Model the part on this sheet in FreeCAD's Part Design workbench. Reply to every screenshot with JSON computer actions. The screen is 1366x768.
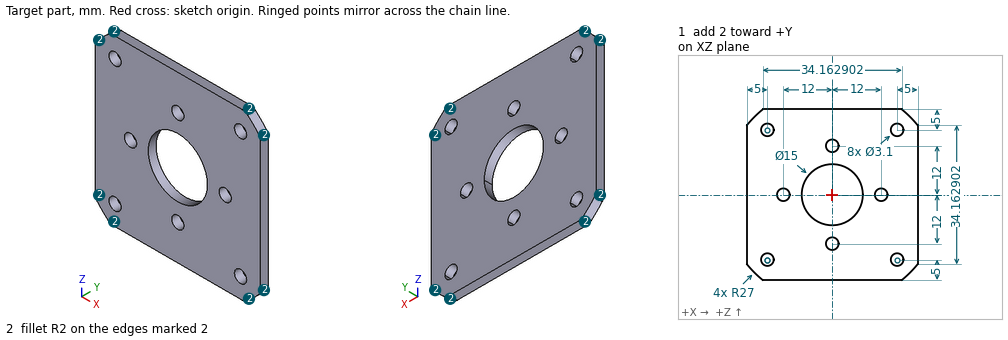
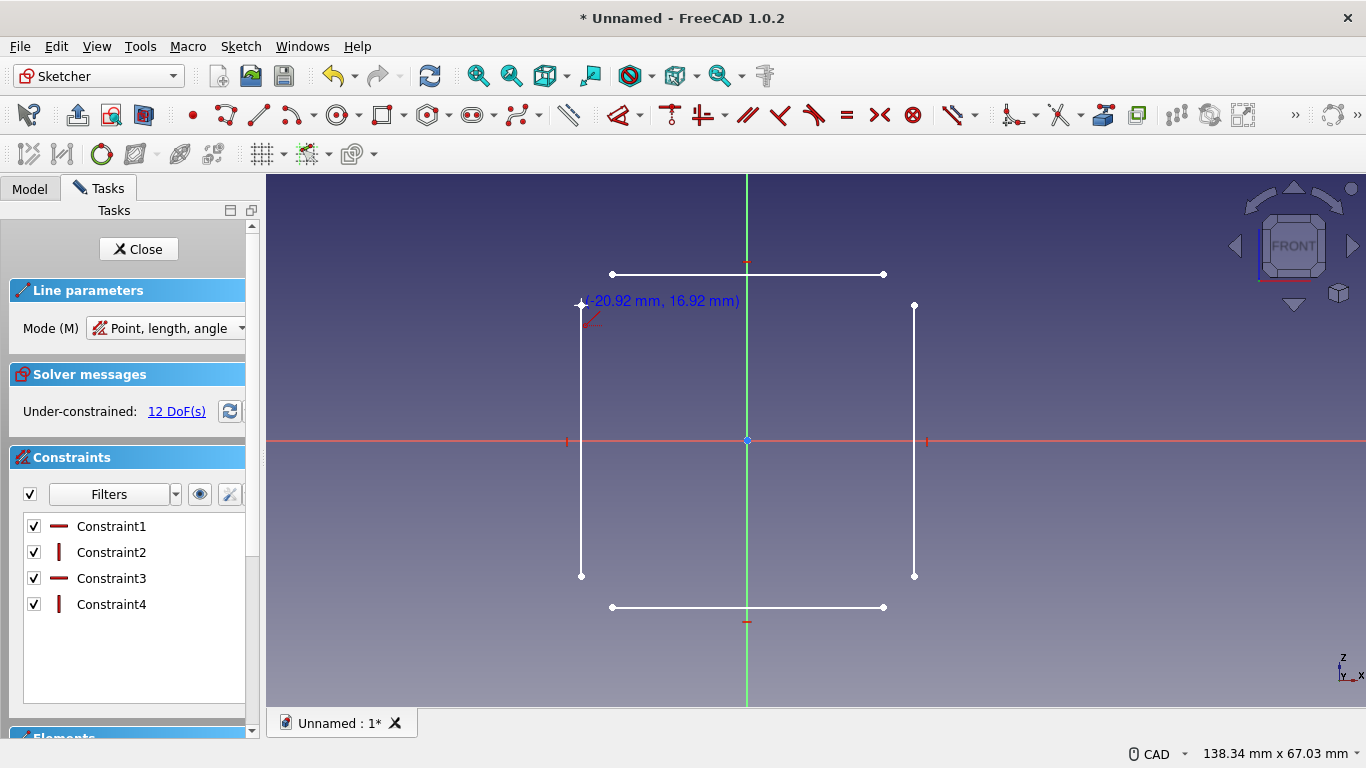
{"action": "left_click", "coordinate": [314, 116]}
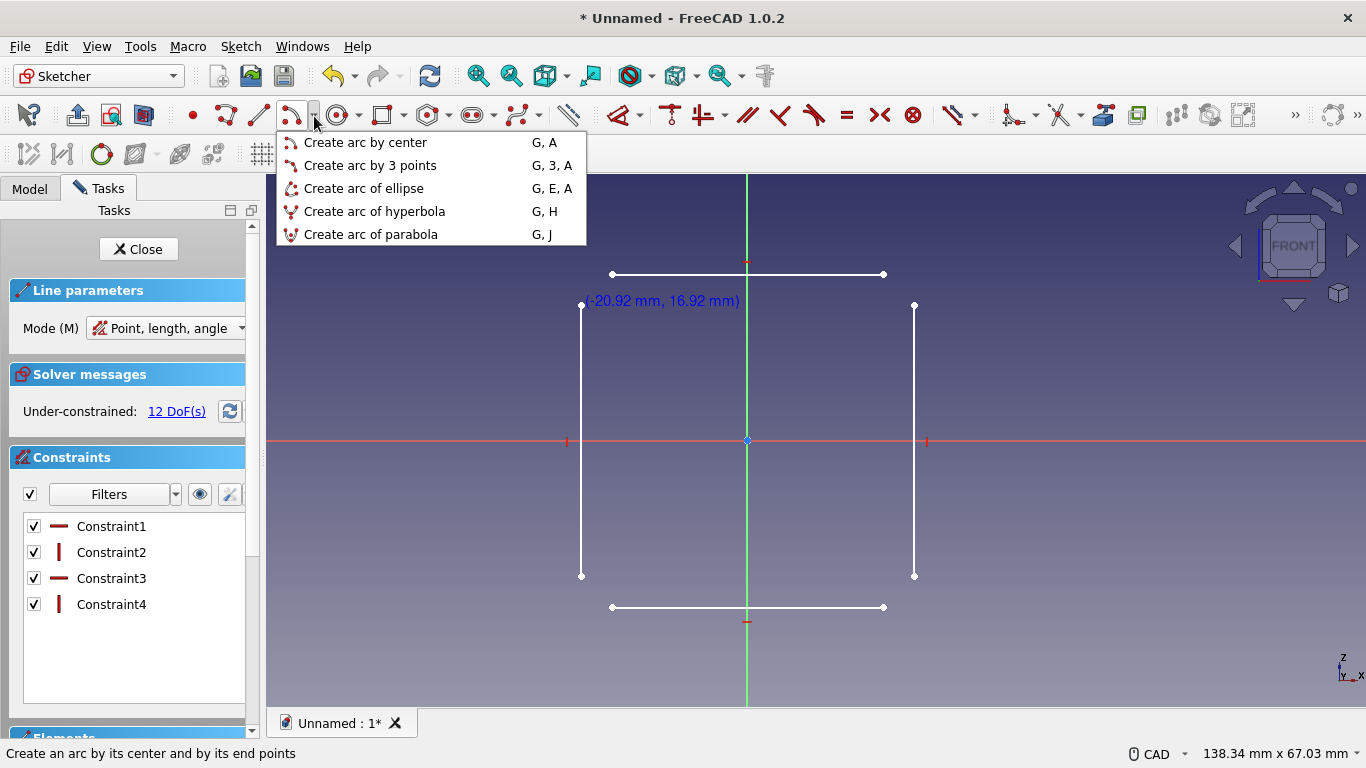
{"action": "left_click", "coordinate": [432, 166]}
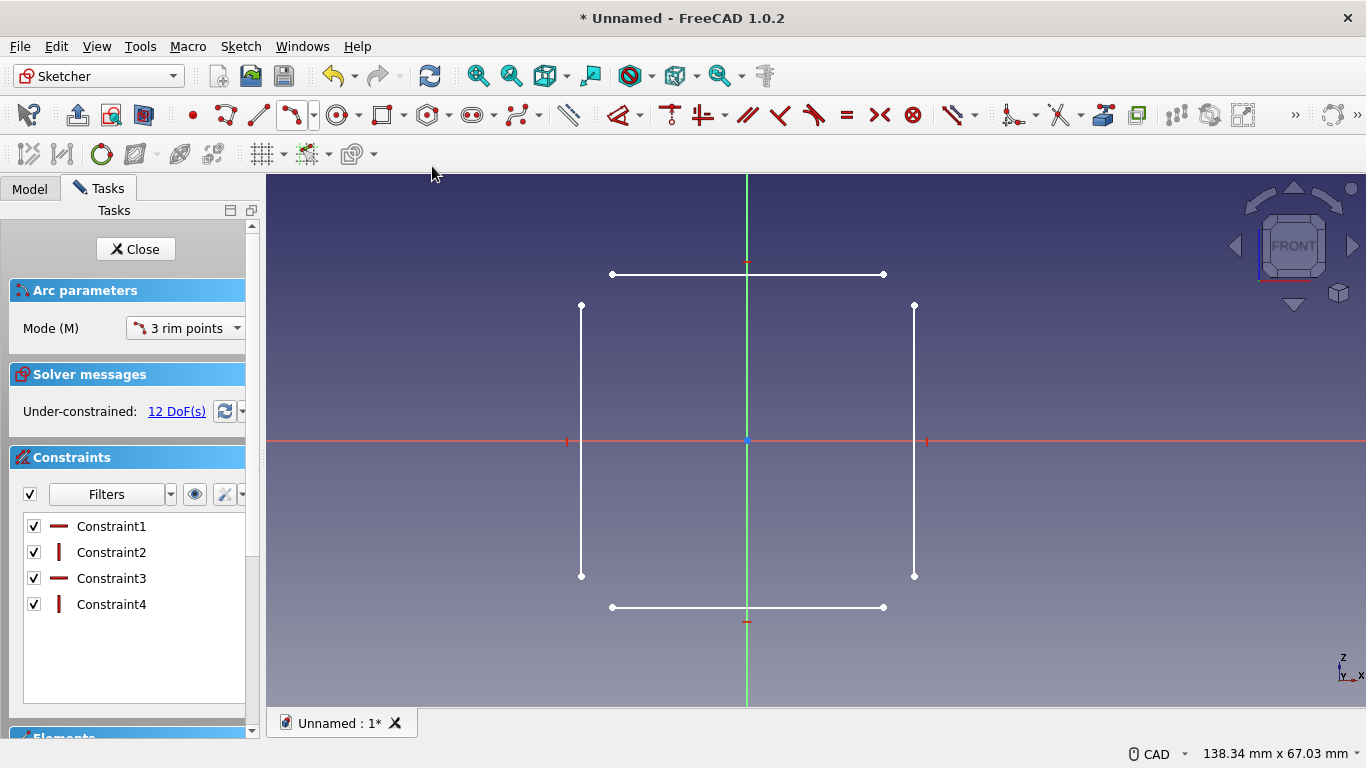
{"action": "left_click", "coordinate": [883, 275]}
{"action": "left_click", "coordinate": [914, 306]}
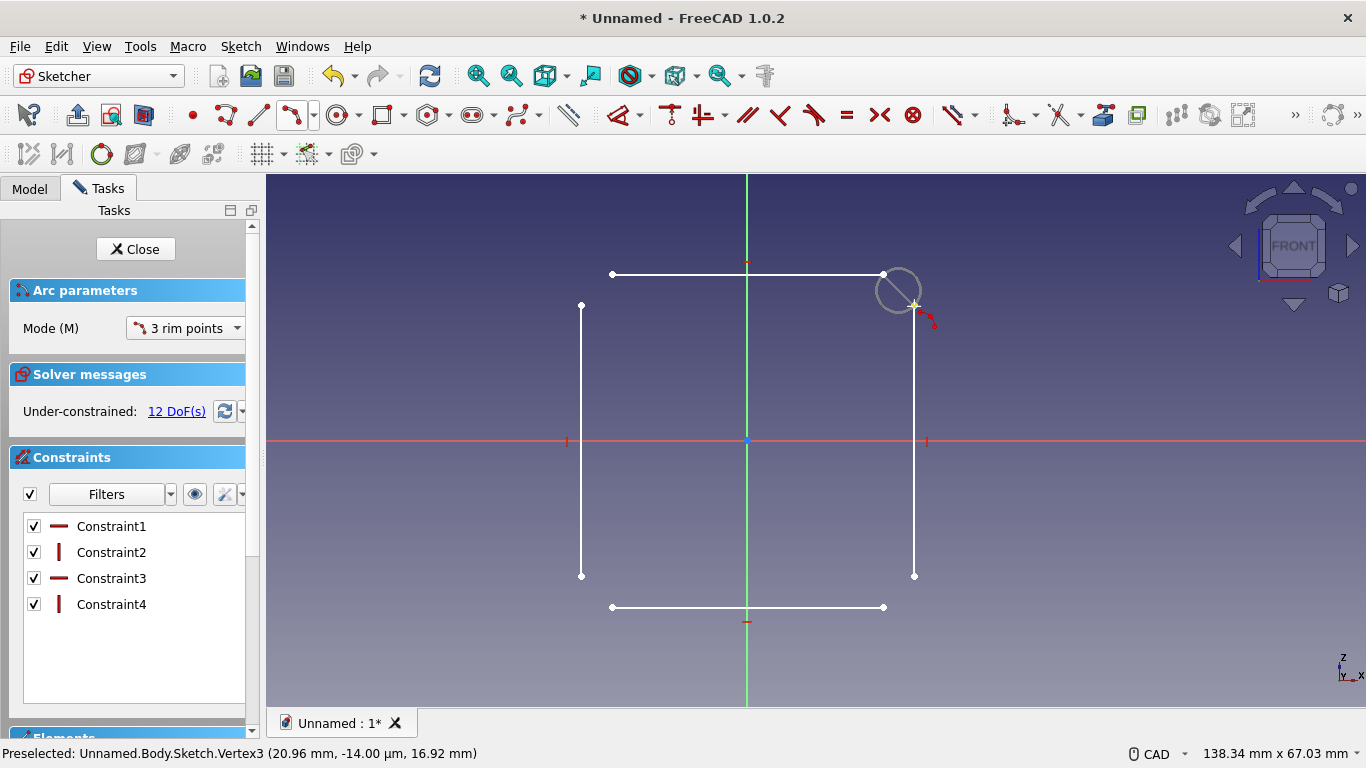
{"action": "scroll", "coordinate": [899, 289], "scroll_direction": "up", "scroll_amount": 14}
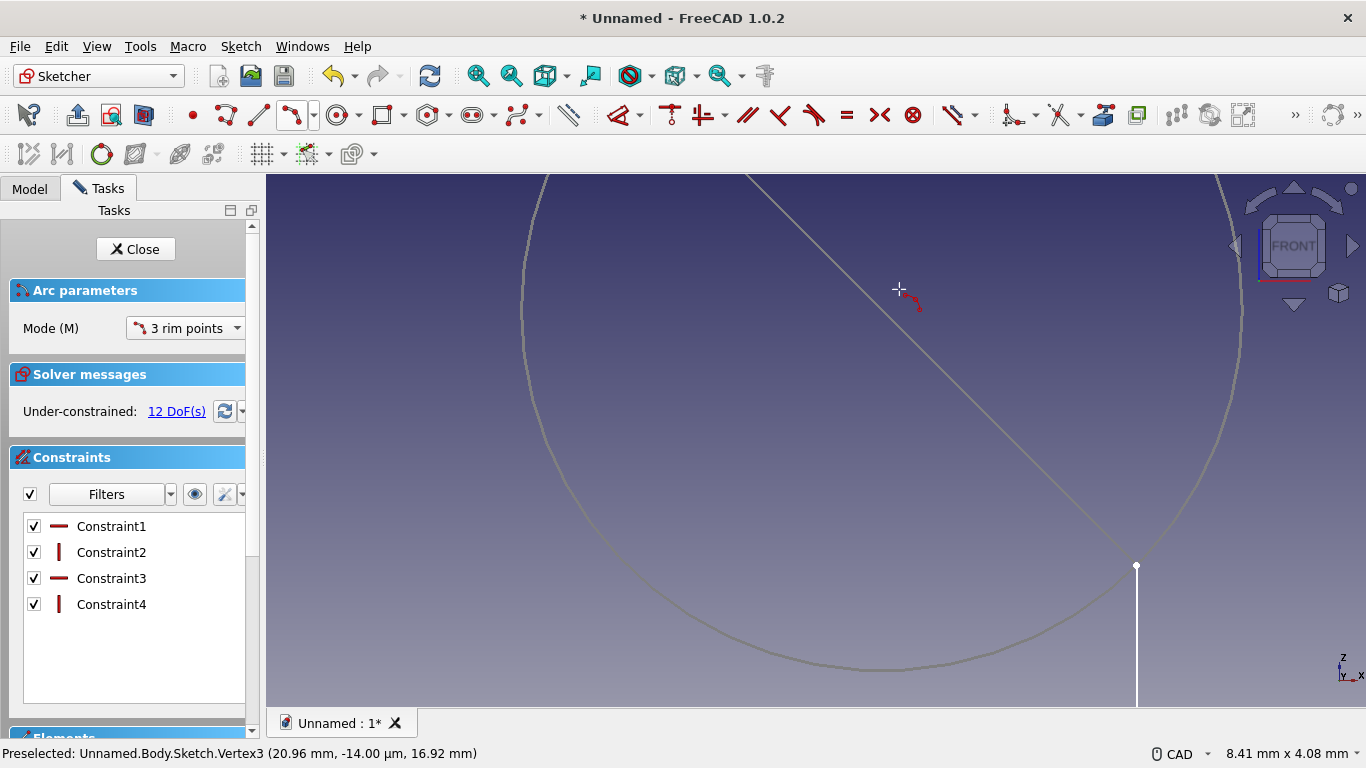
{"action": "left_click", "coordinate": [892, 281]}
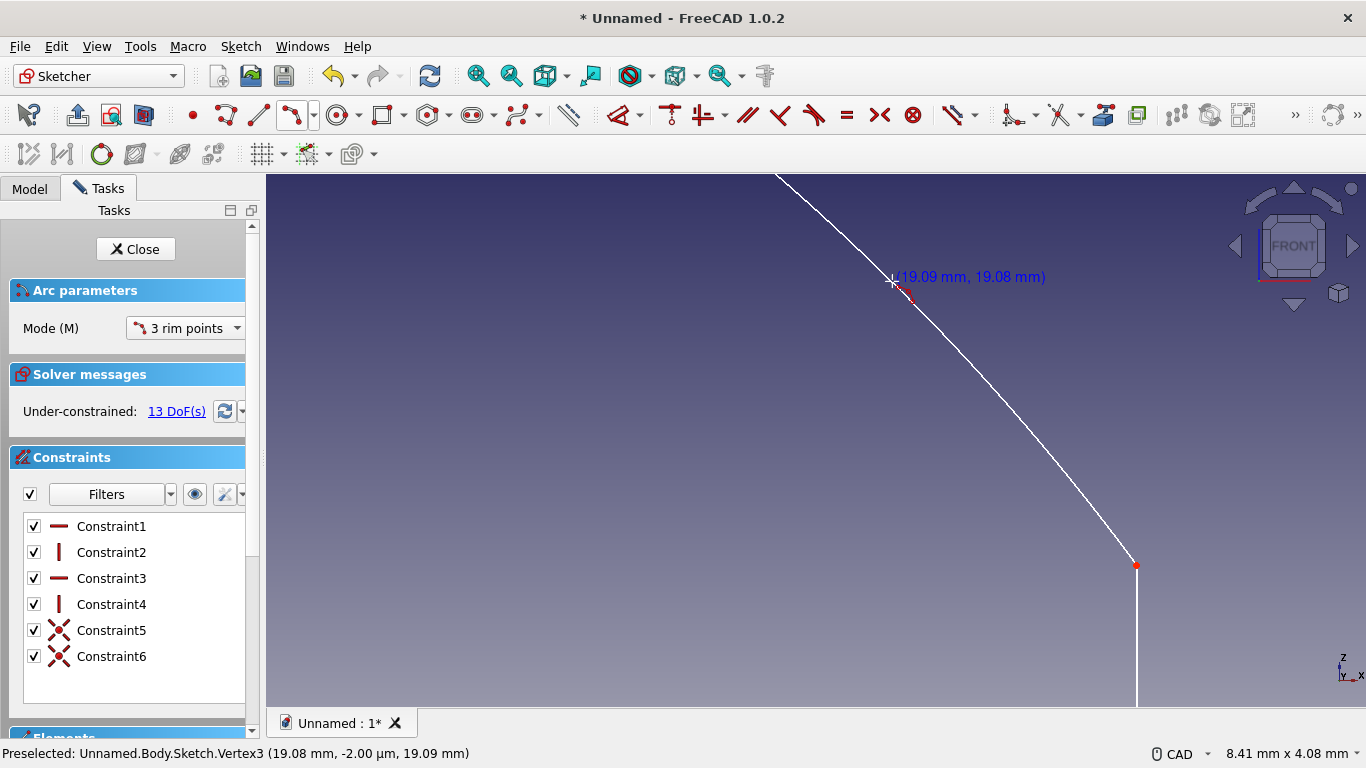
{"action": "scroll", "coordinate": [900, 289], "scroll_direction": "down", "scroll_amount": 14}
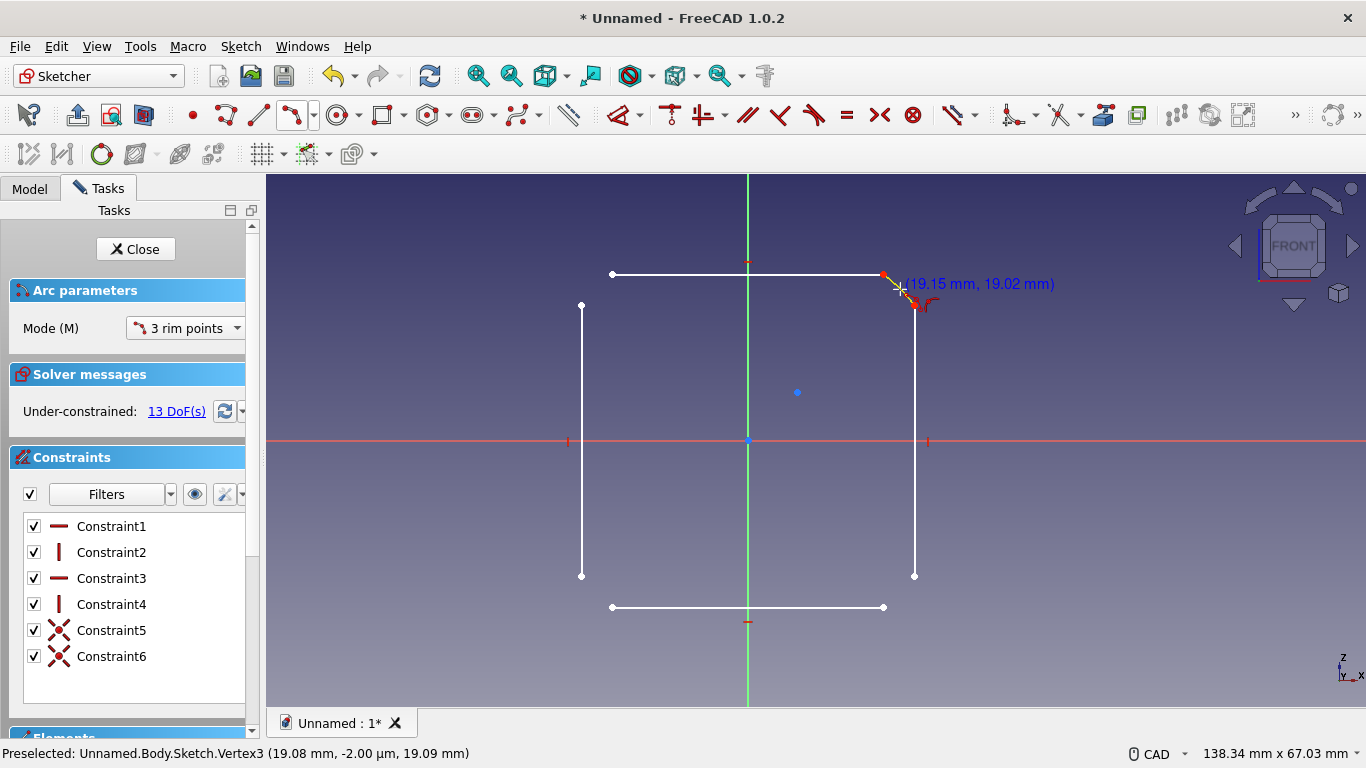
{"action": "left_click", "coordinate": [915, 577]}
{"action": "left_click", "coordinate": [884, 608]}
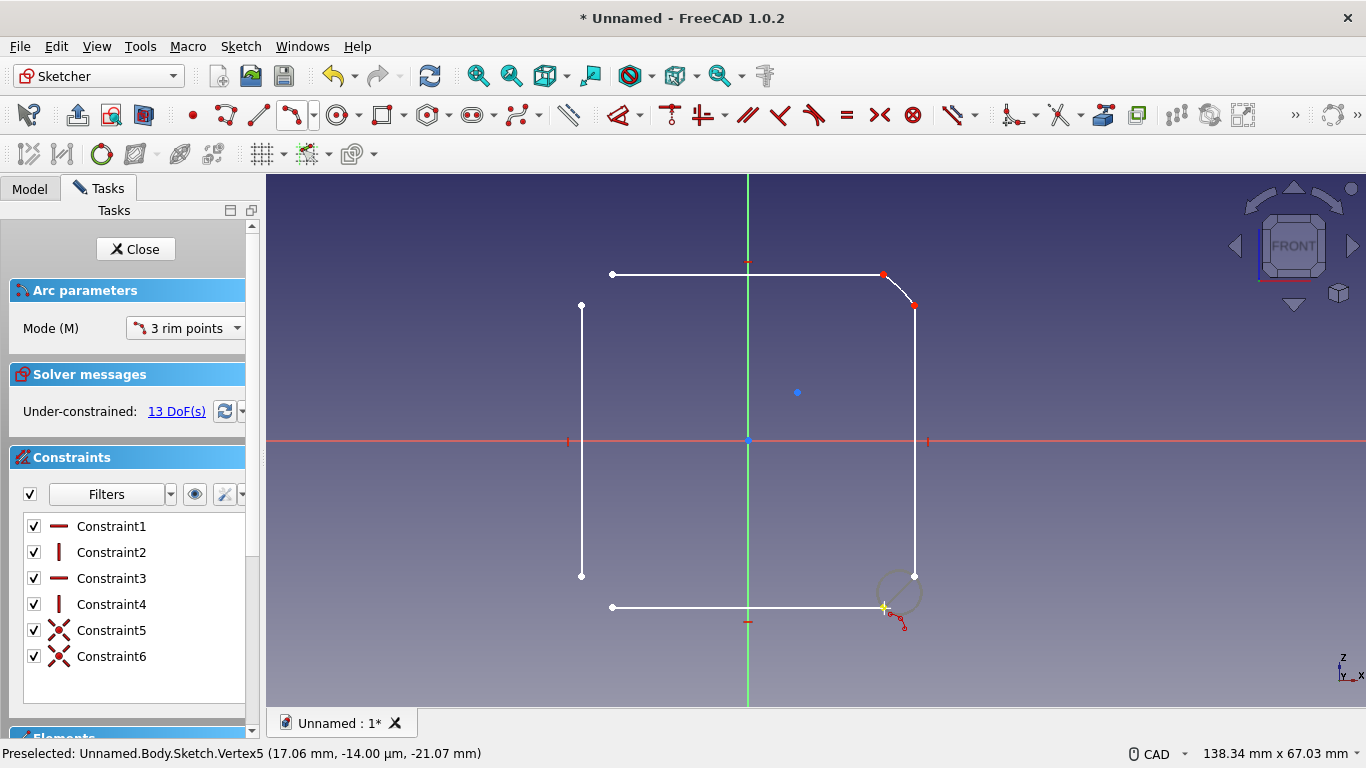
{"action": "scroll", "coordinate": [900, 592], "scroll_direction": "up", "scroll_amount": 14}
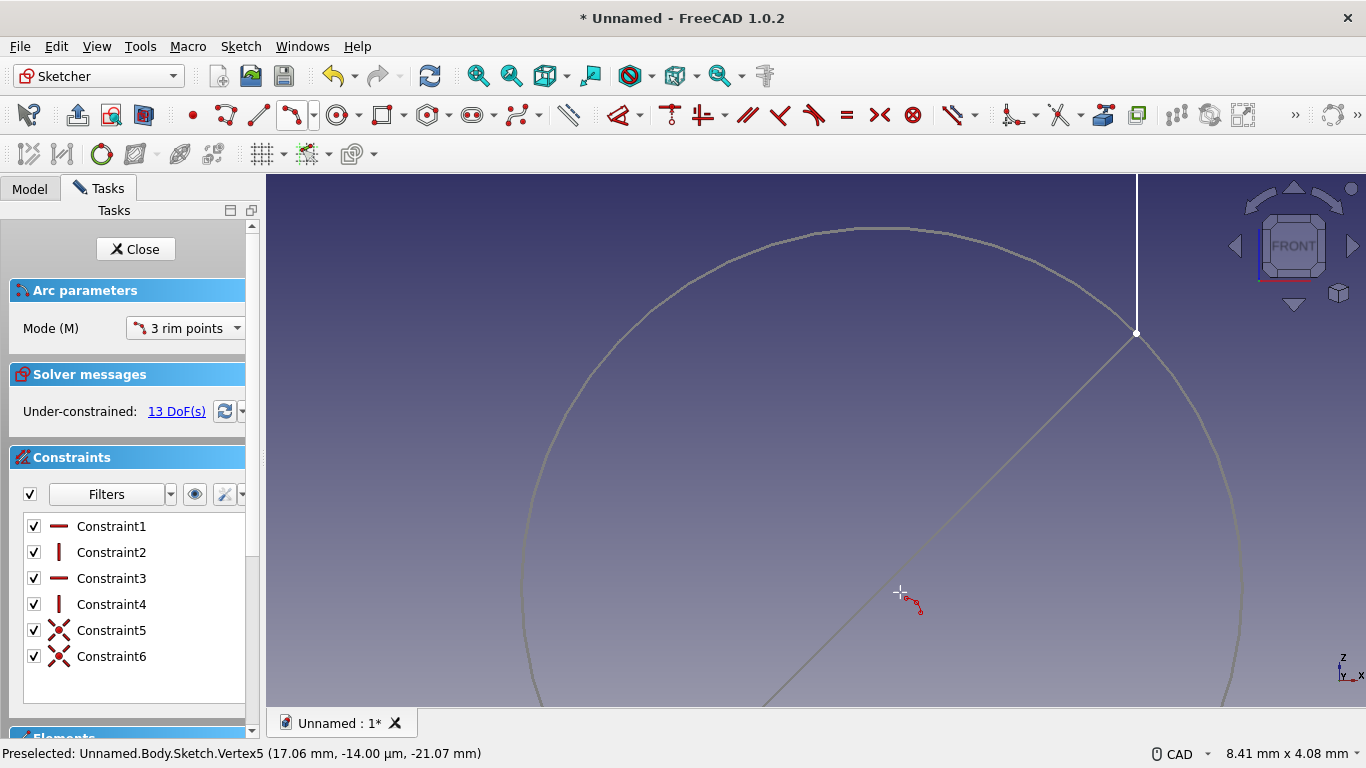
{"action": "left_click", "coordinate": [892, 585]}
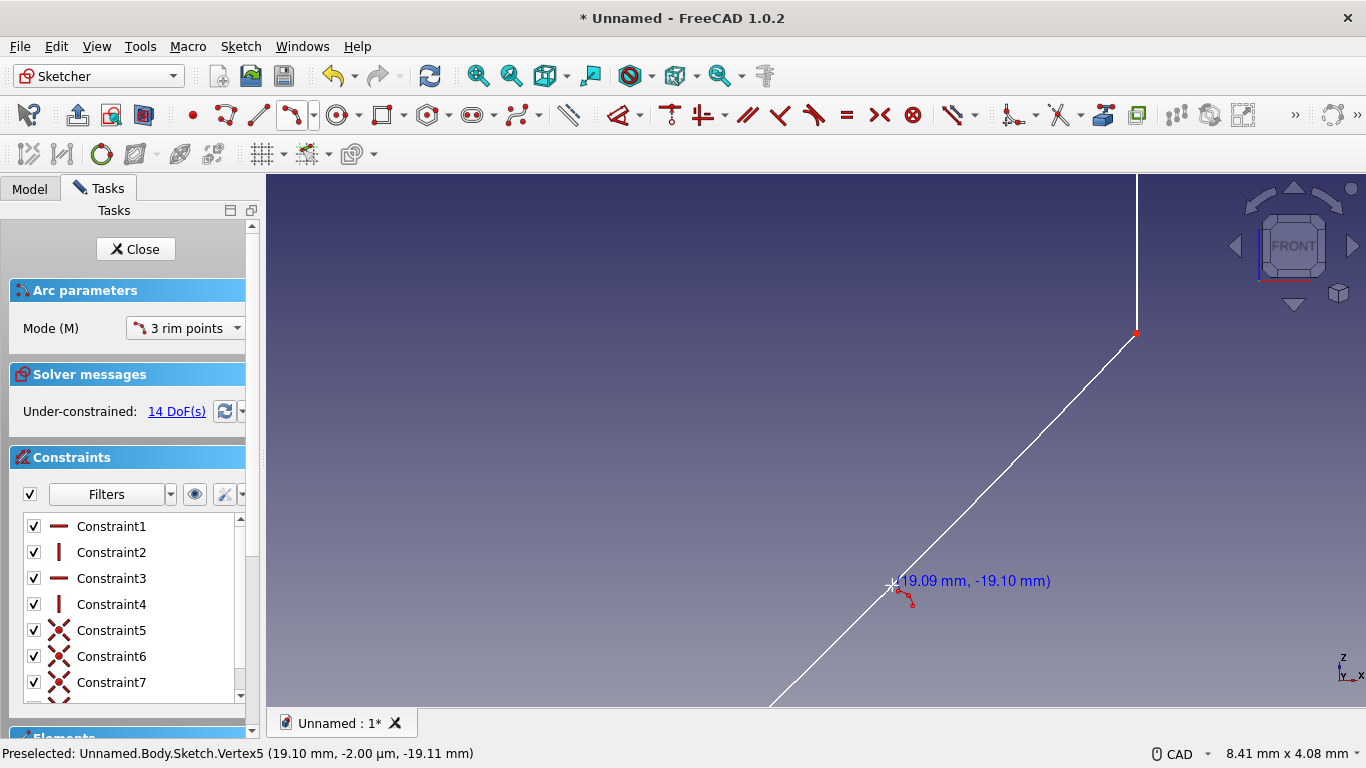
{"action": "scroll", "coordinate": [900, 593], "scroll_direction": "down", "scroll_amount": 14}